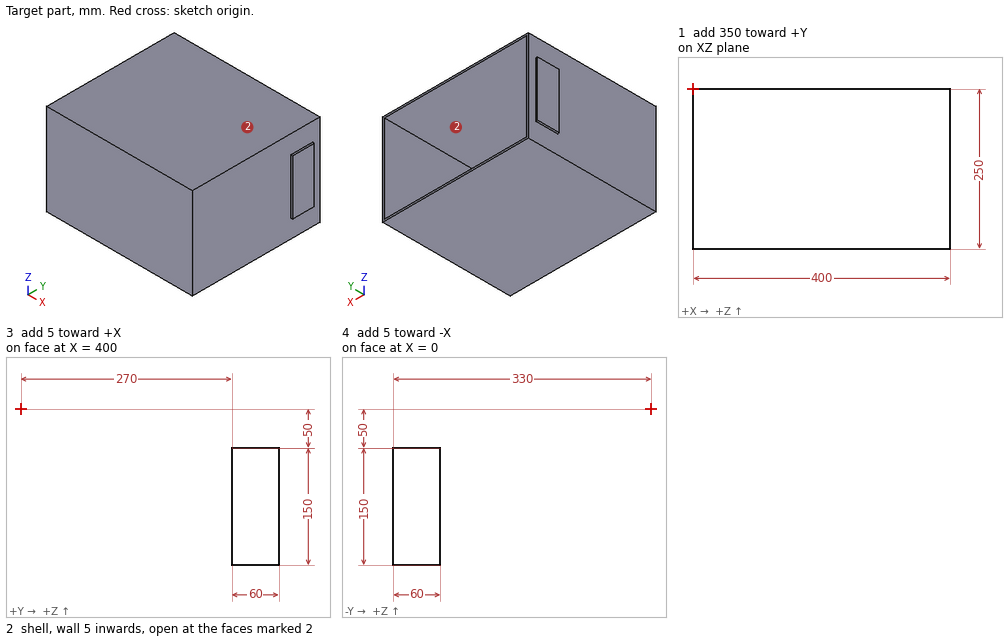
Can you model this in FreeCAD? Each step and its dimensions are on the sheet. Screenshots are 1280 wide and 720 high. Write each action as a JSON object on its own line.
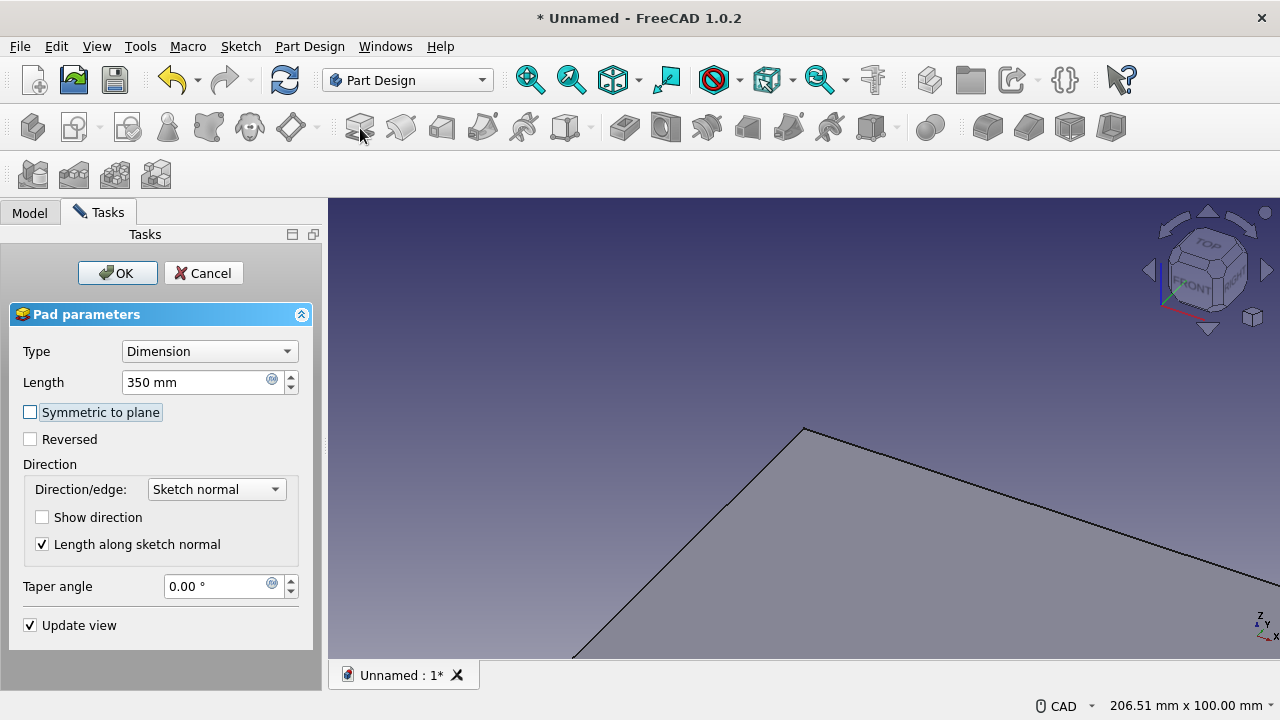
{"action": "left_click", "coordinate": [31, 439]}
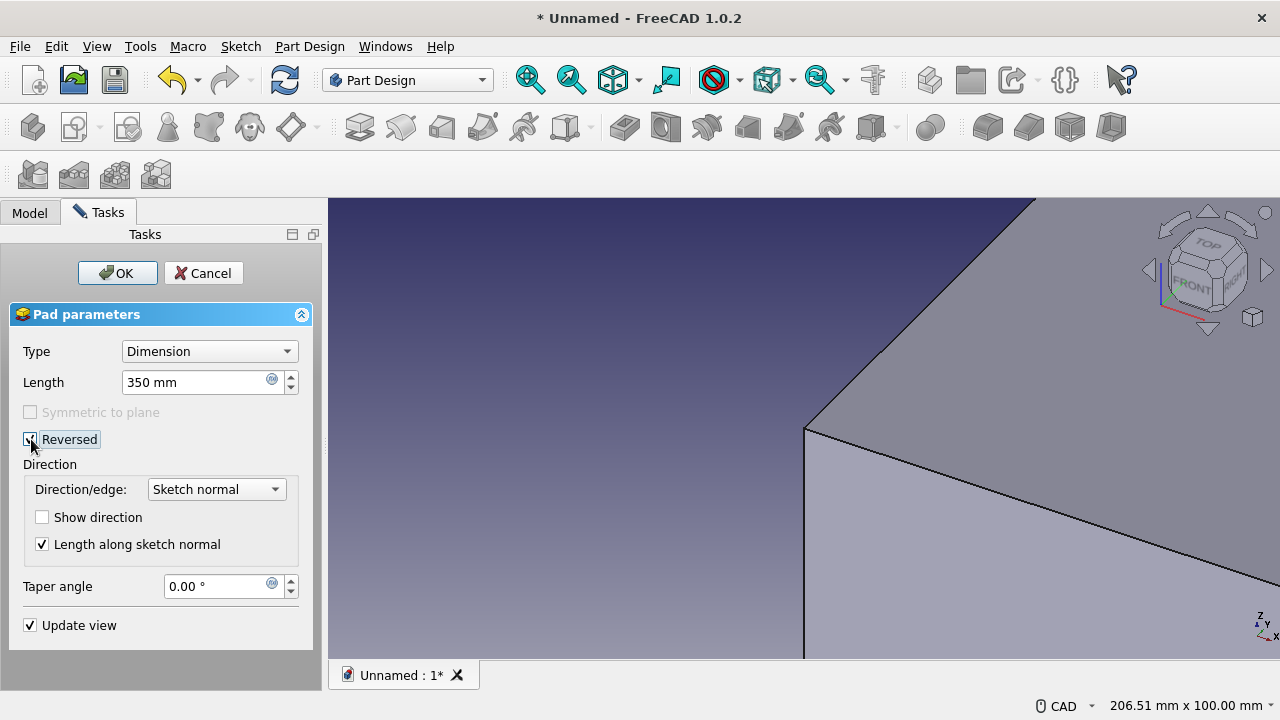
{"action": "left_click", "coordinate": [118, 273]}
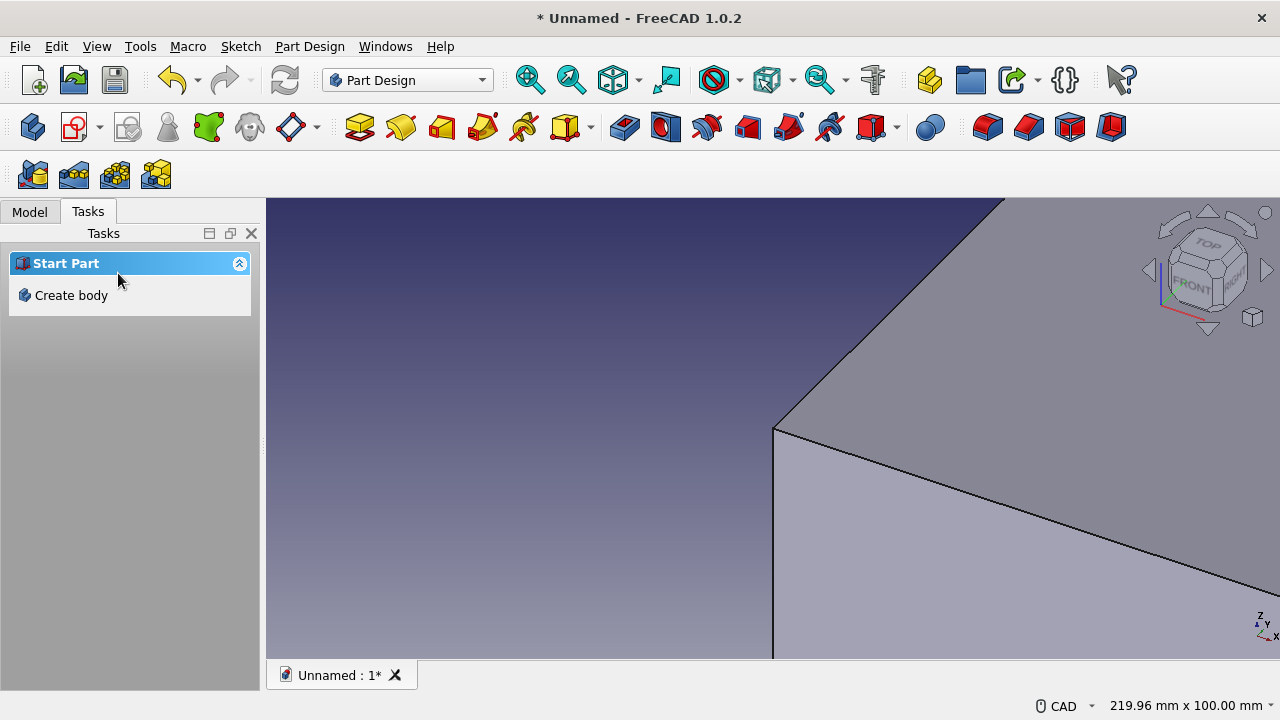
{"action": "key", "text": "v f"}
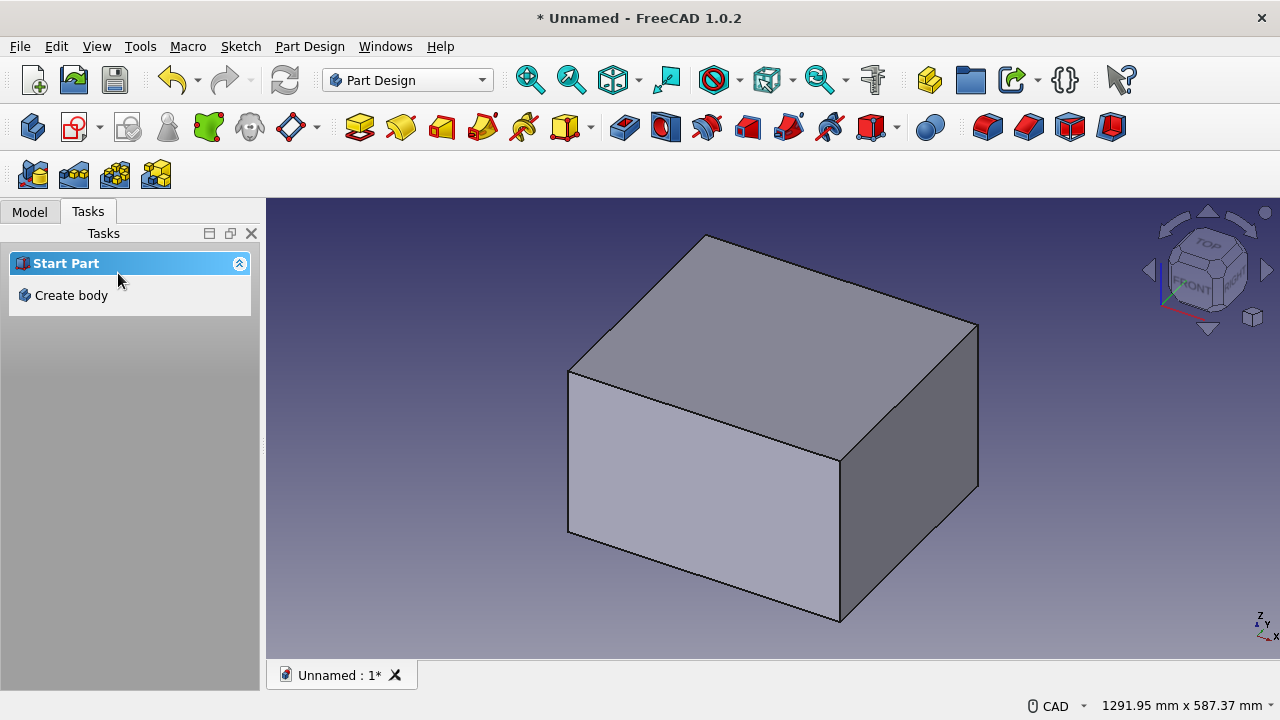
{"action": "key", "text": "0"}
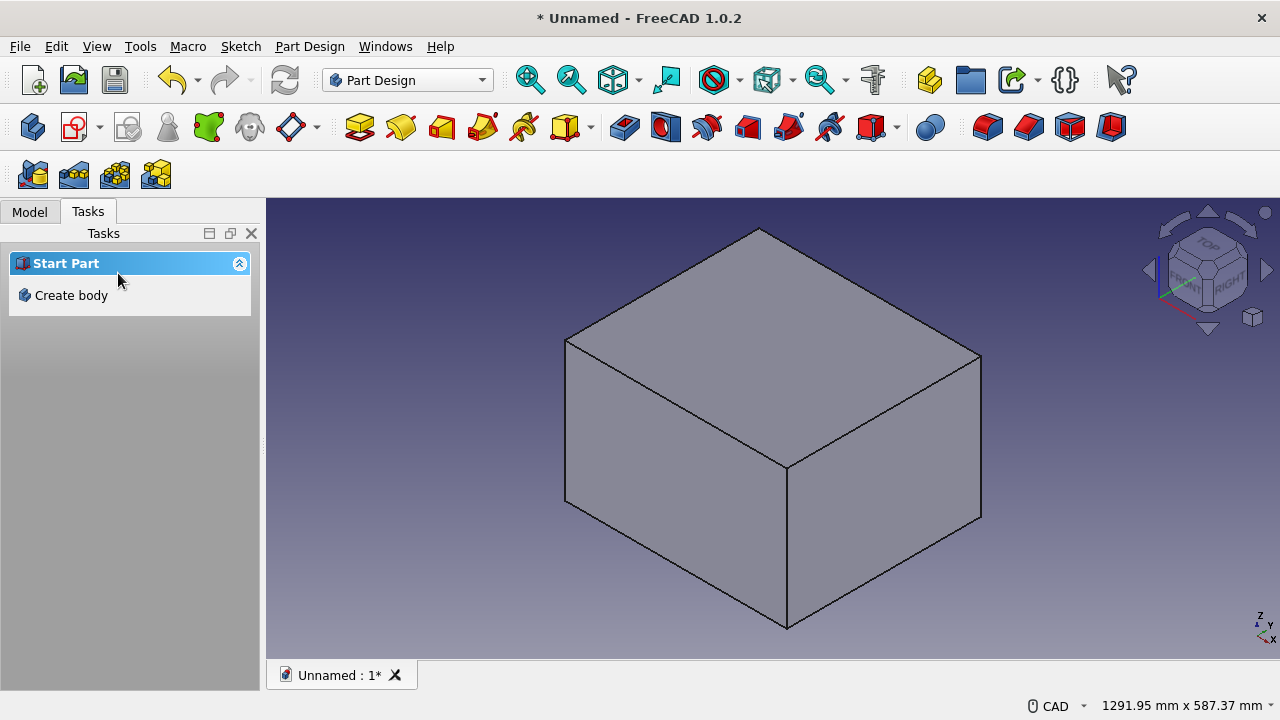
{"action": "key", "text": "2"}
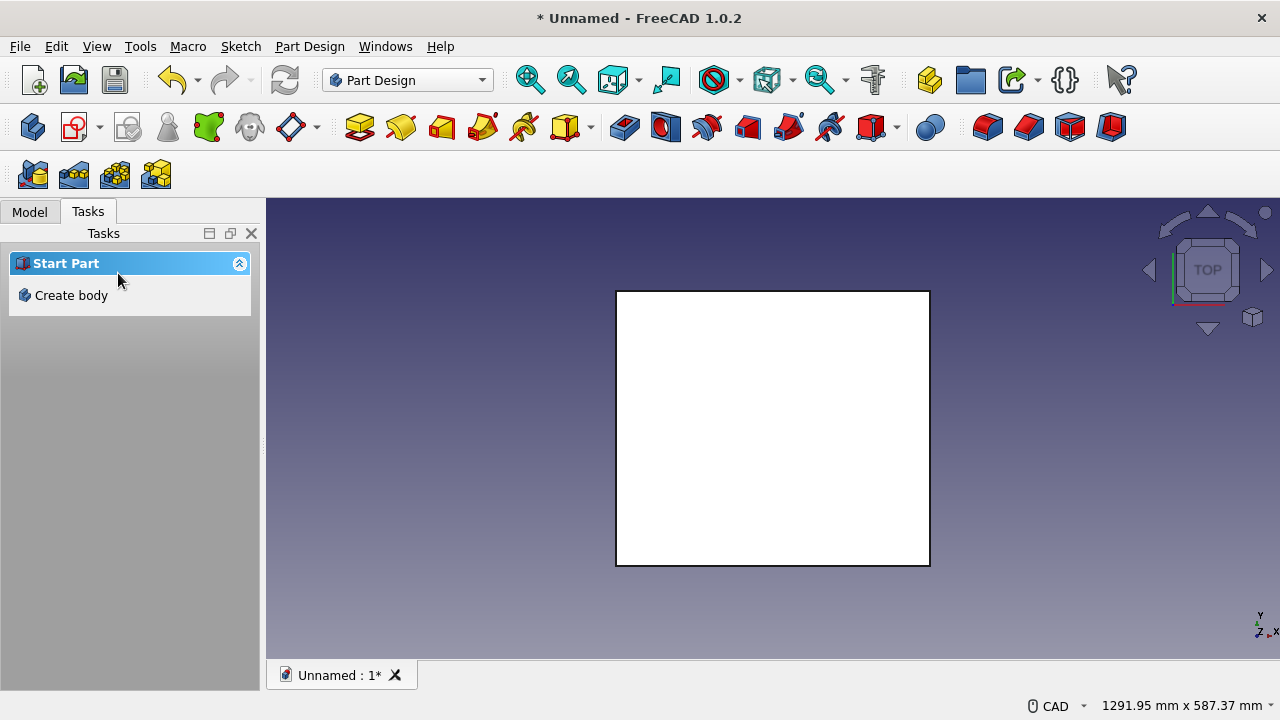
{"action": "key", "text": "1"}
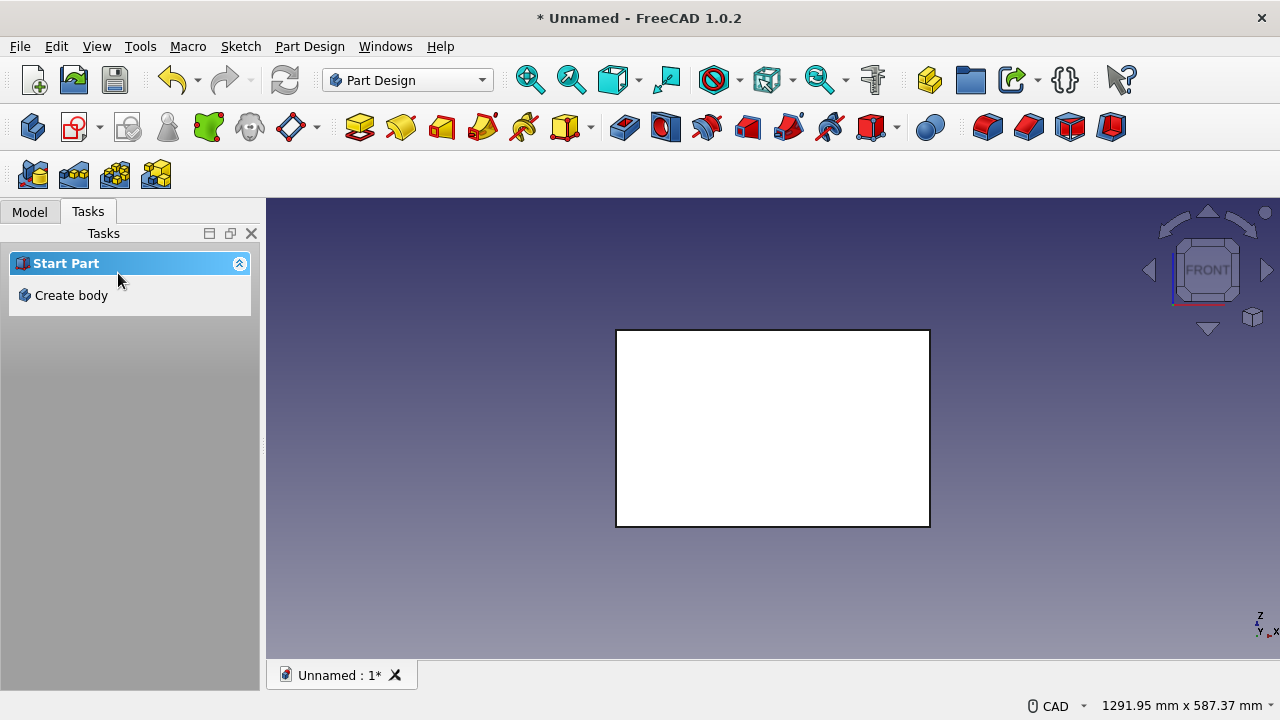
{"action": "left_click", "coordinate": [531, 80]}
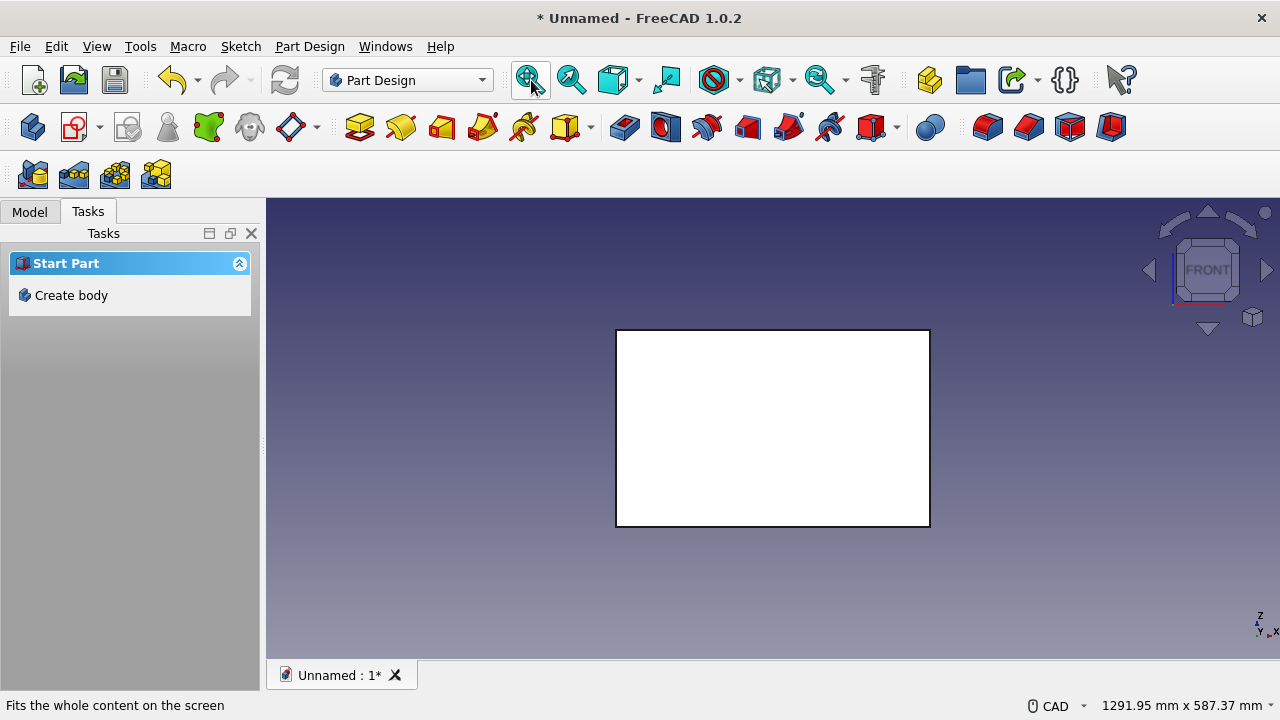
{"action": "key", "text": "3"}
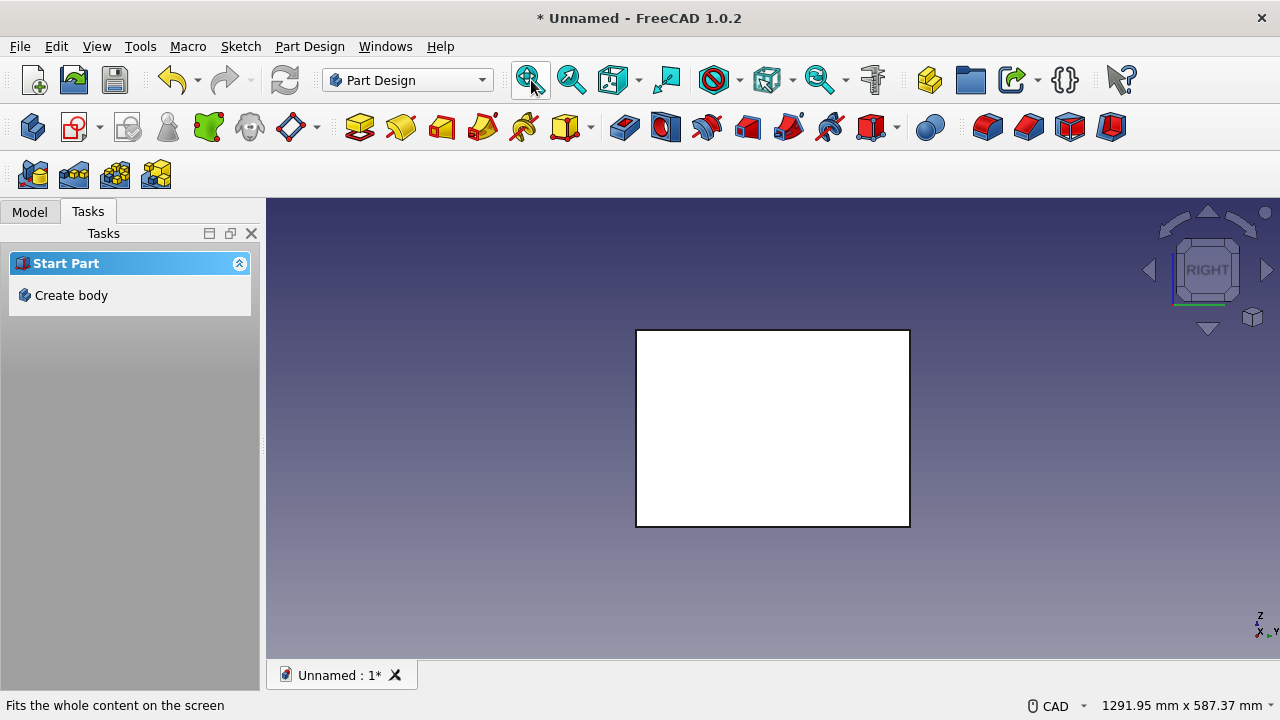
{"action": "left_click", "coordinate": [531, 80]}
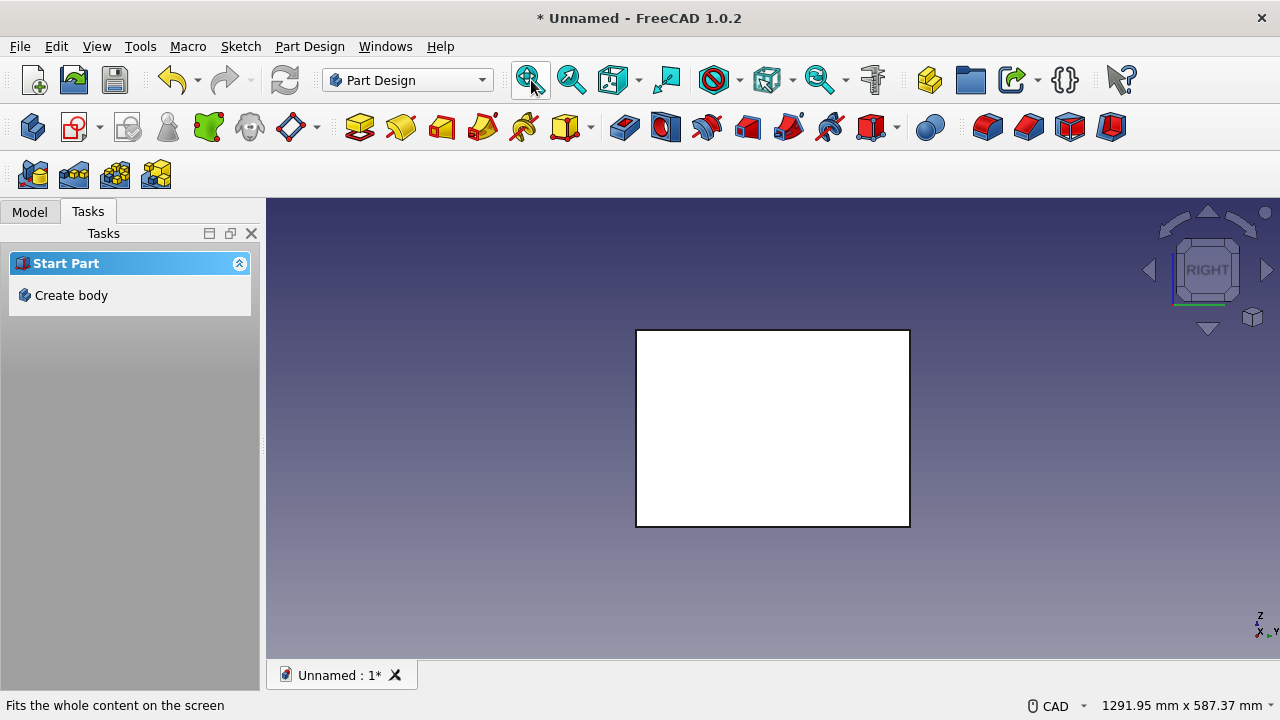
{"action": "key", "text": "5"}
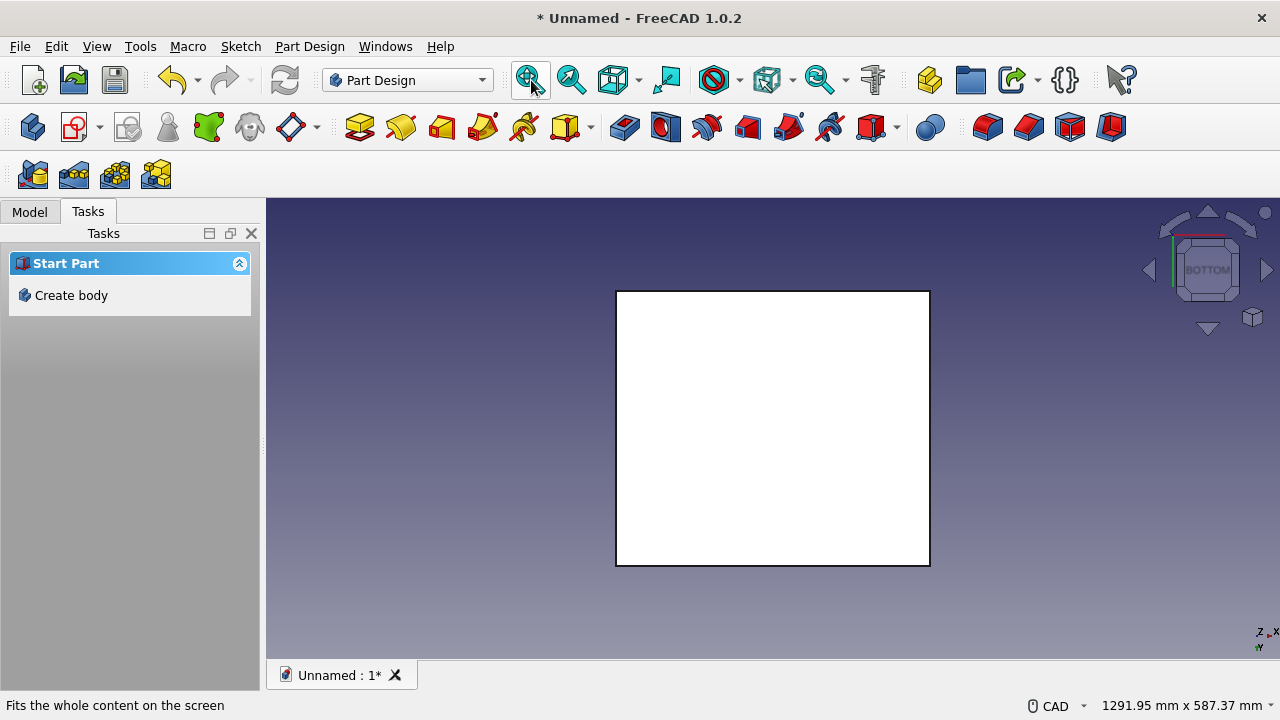
{"action": "key", "text": "4"}